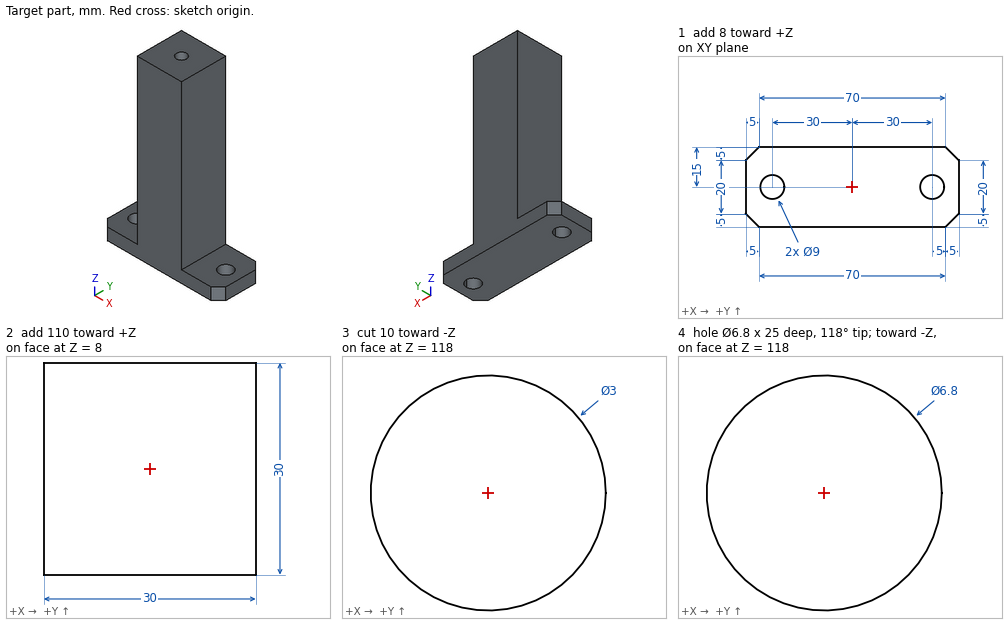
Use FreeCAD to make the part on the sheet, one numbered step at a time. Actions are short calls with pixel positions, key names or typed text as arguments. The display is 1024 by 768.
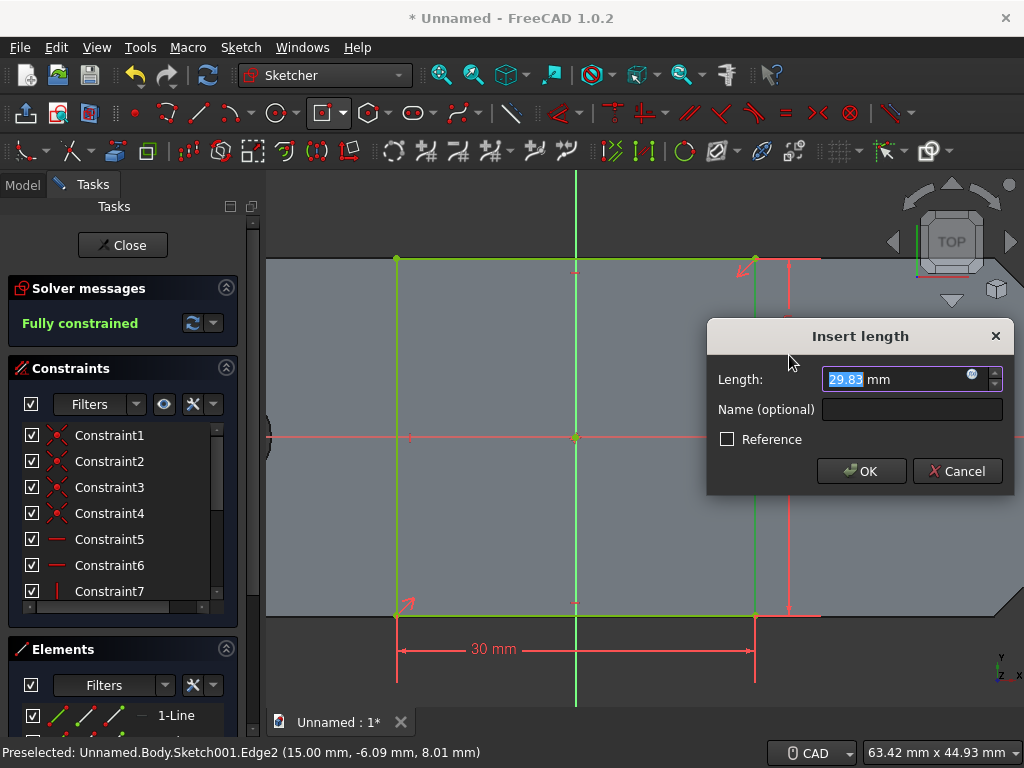
text(30)
key(Return)
key(Escape)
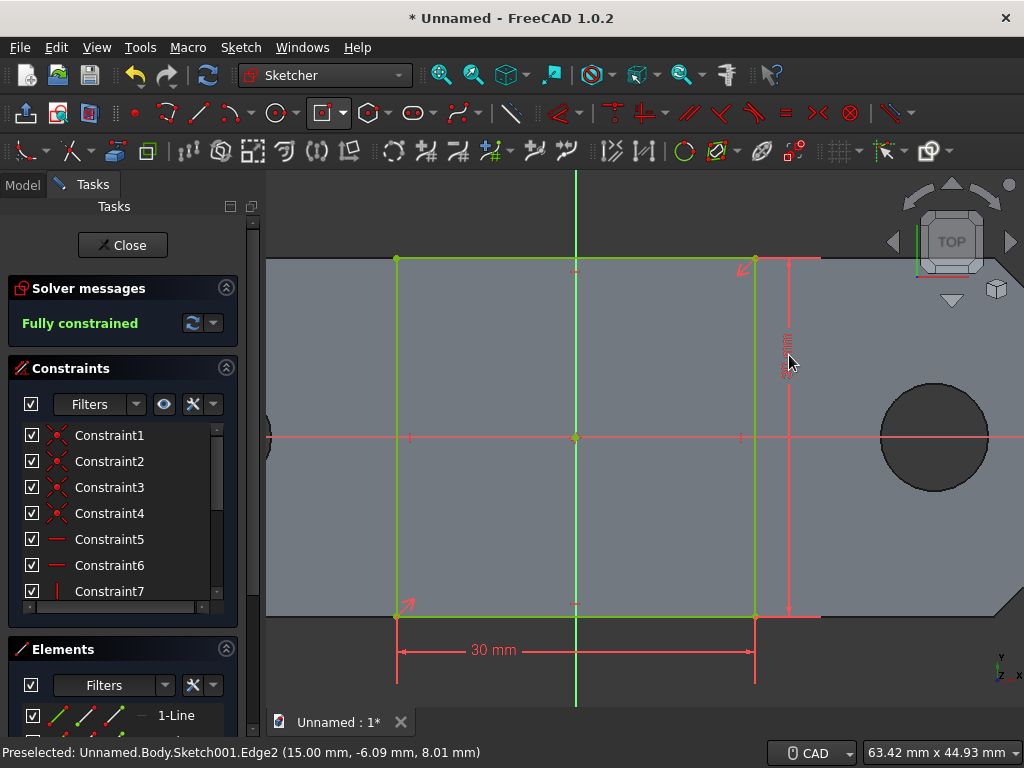
click(123, 245)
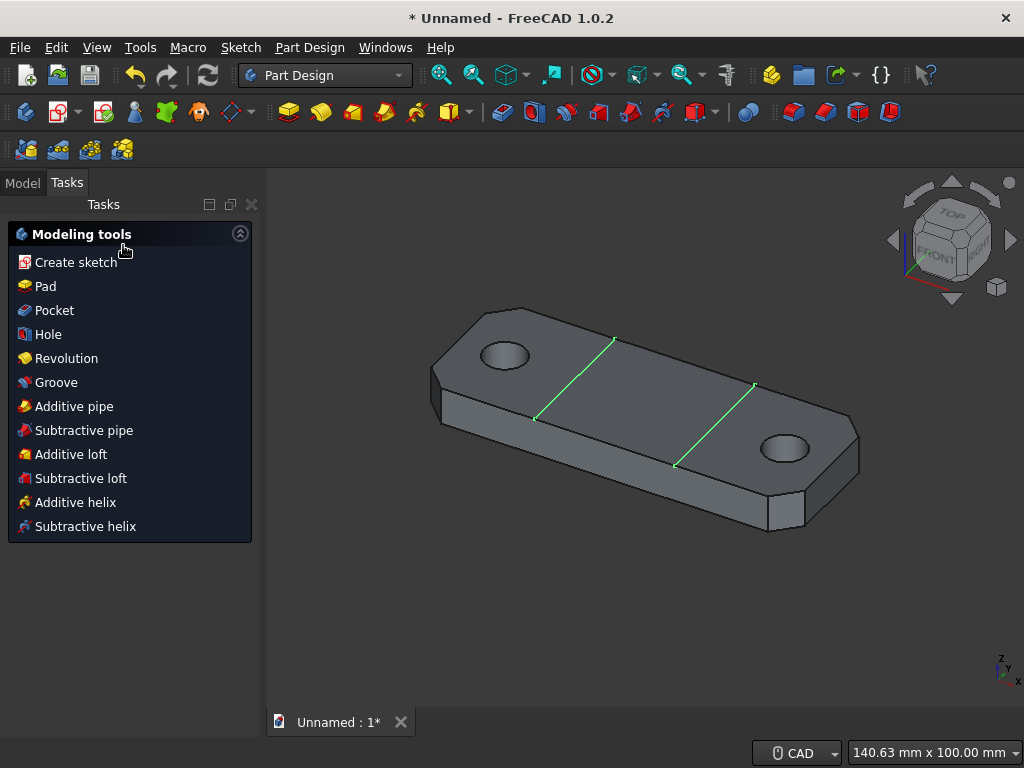
click(290, 112)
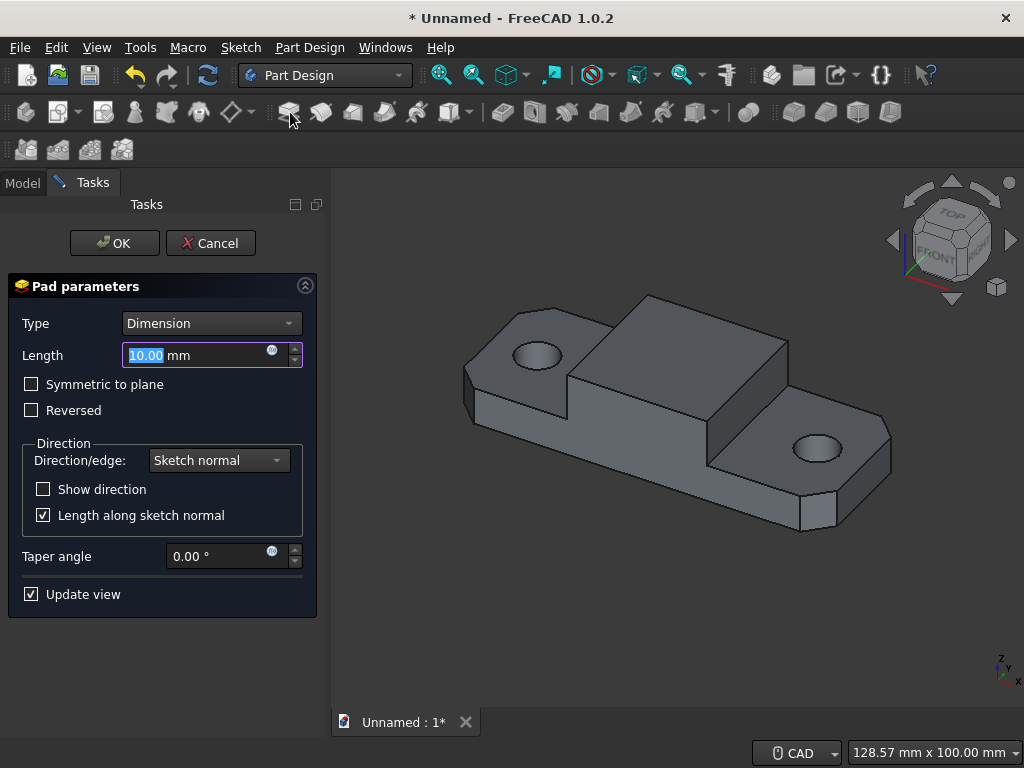
text(110)
key(Tab)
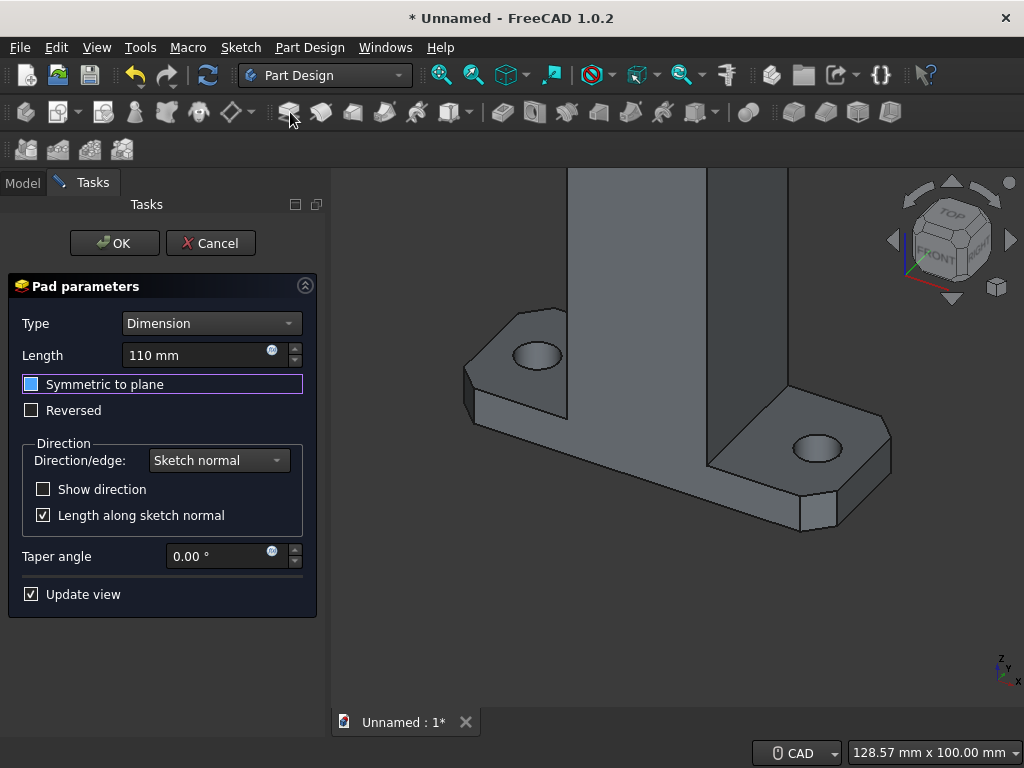
click(115, 243)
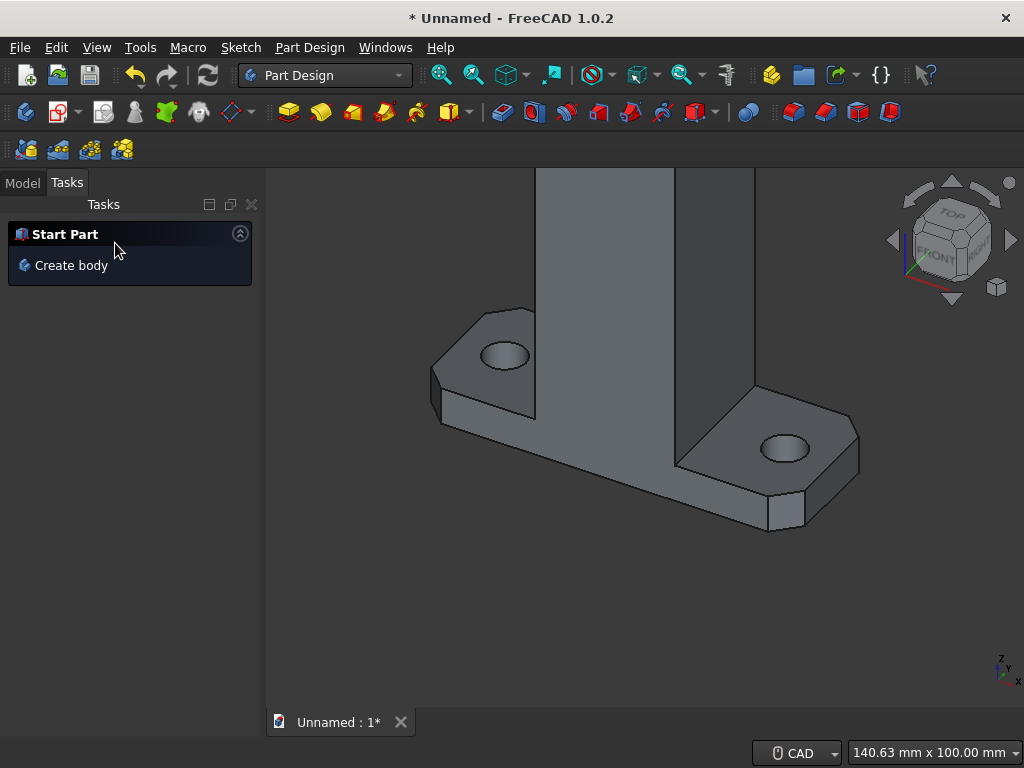
click(442, 76)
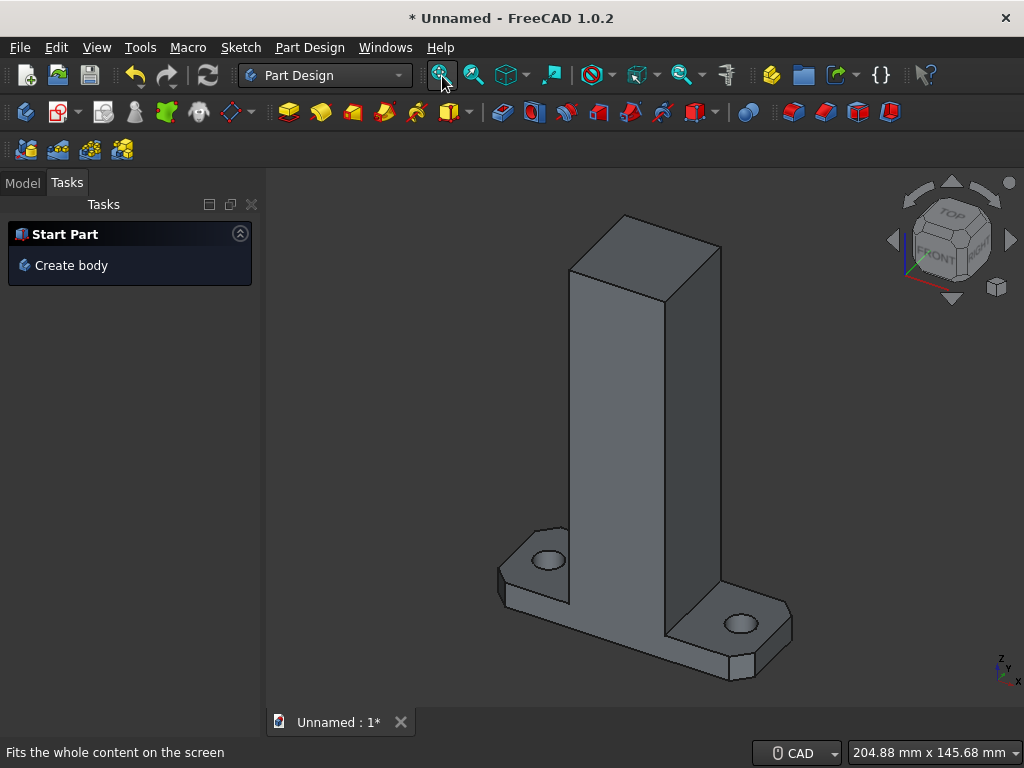
click(645, 258)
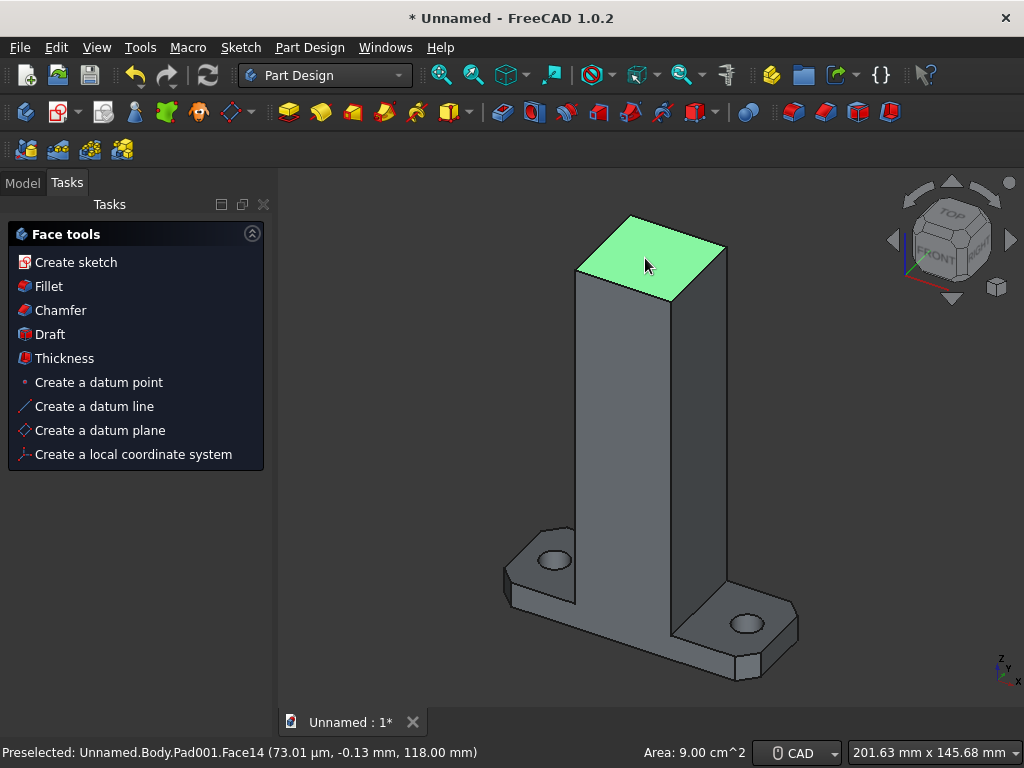
click(58, 112)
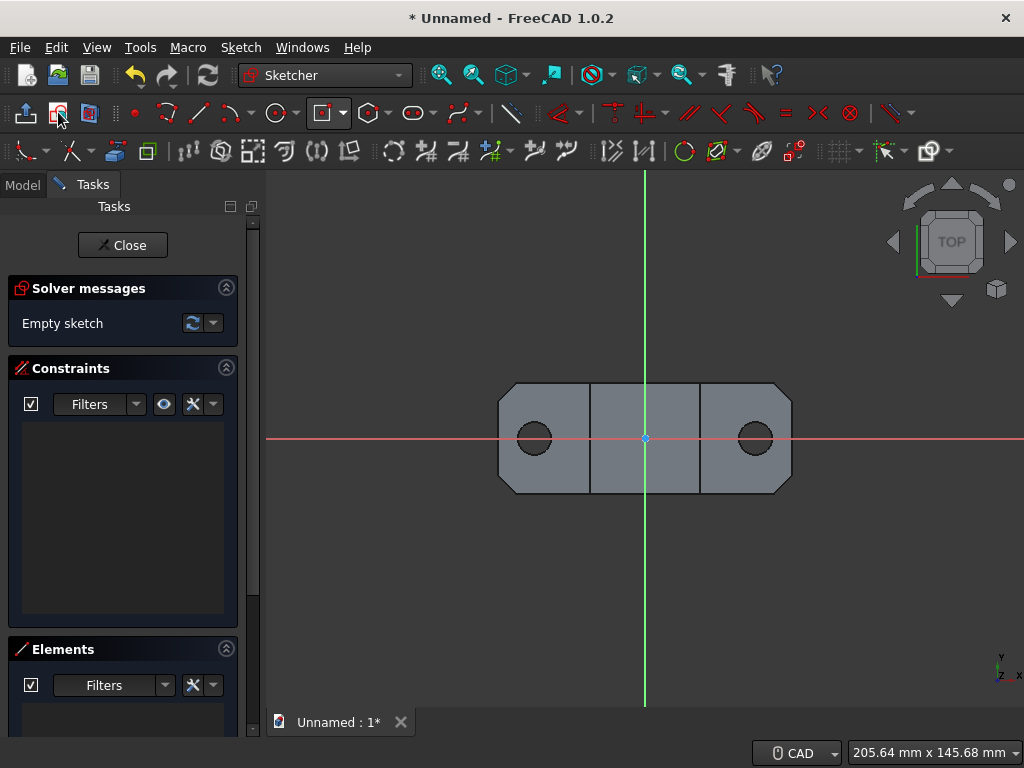
scroll(649, 438, up, 15)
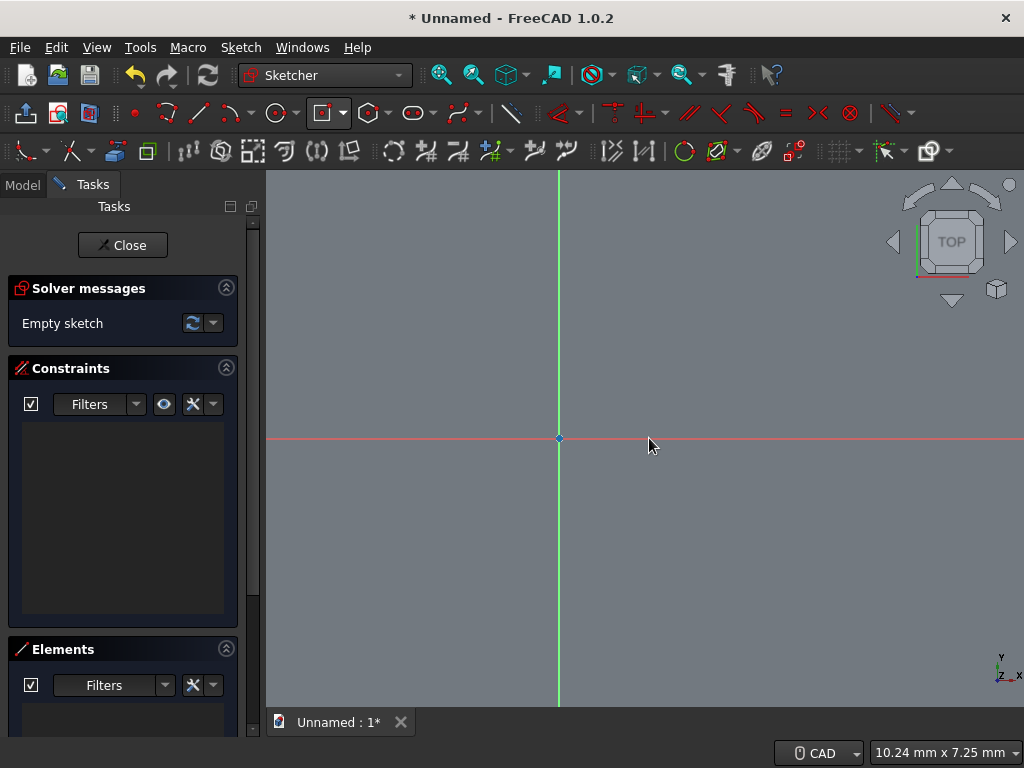
scroll(523, 439, up, 2)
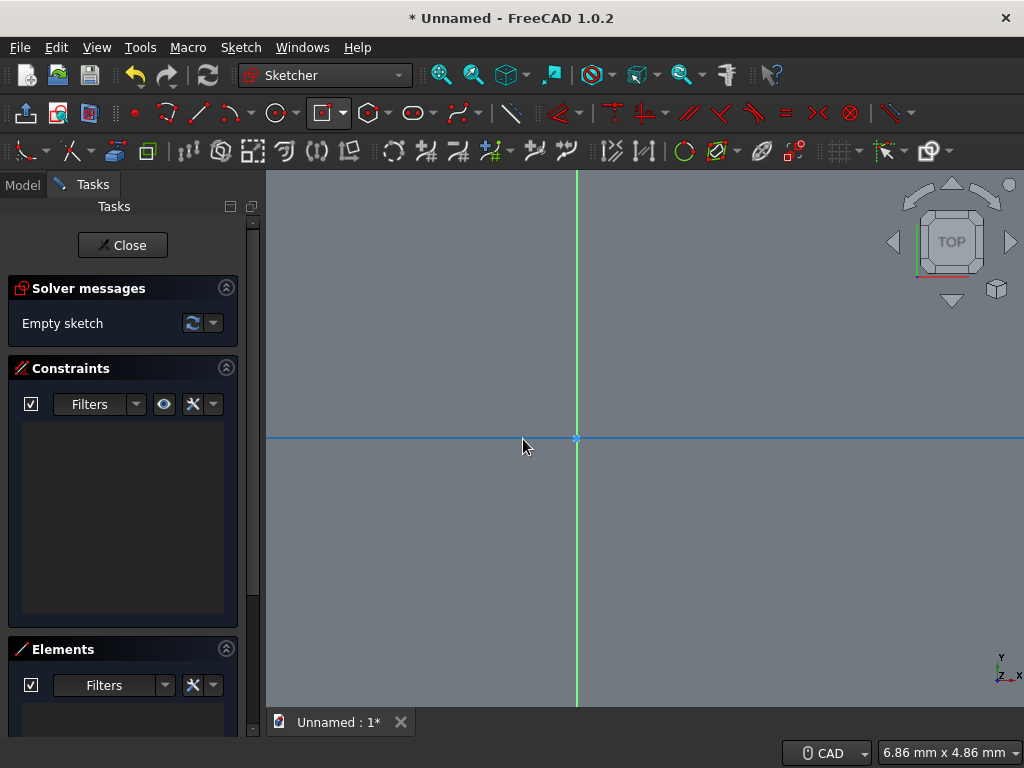
click(276, 114)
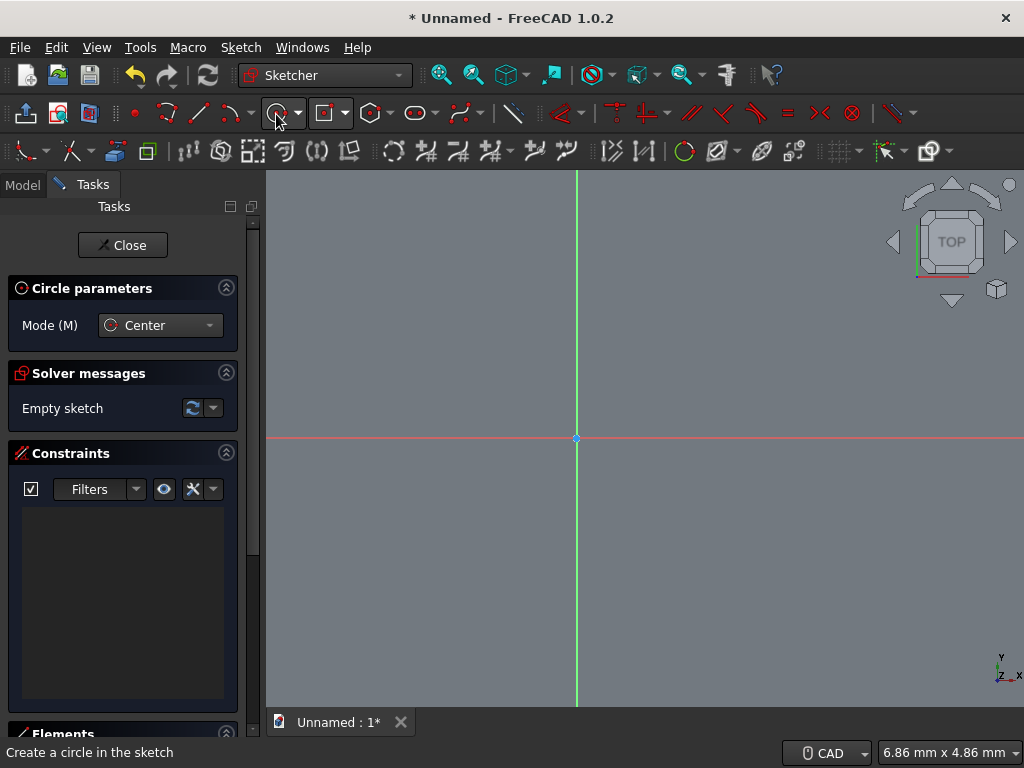
click(577, 438)
click(694, 321)
key(Escape)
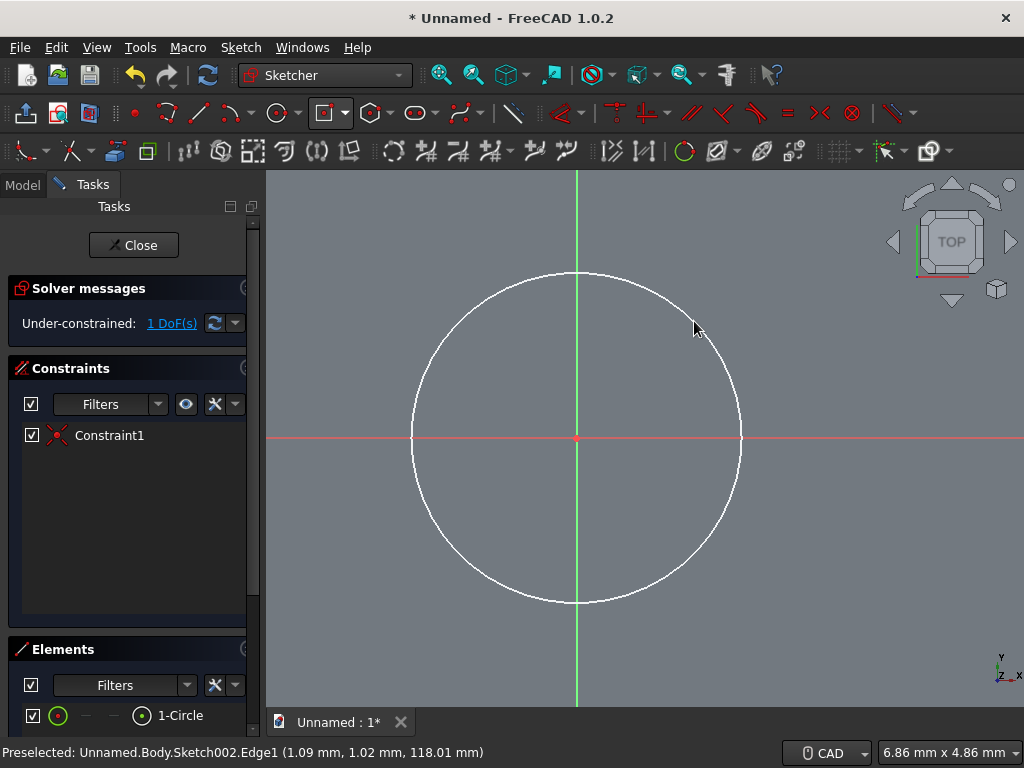
click(560, 114)